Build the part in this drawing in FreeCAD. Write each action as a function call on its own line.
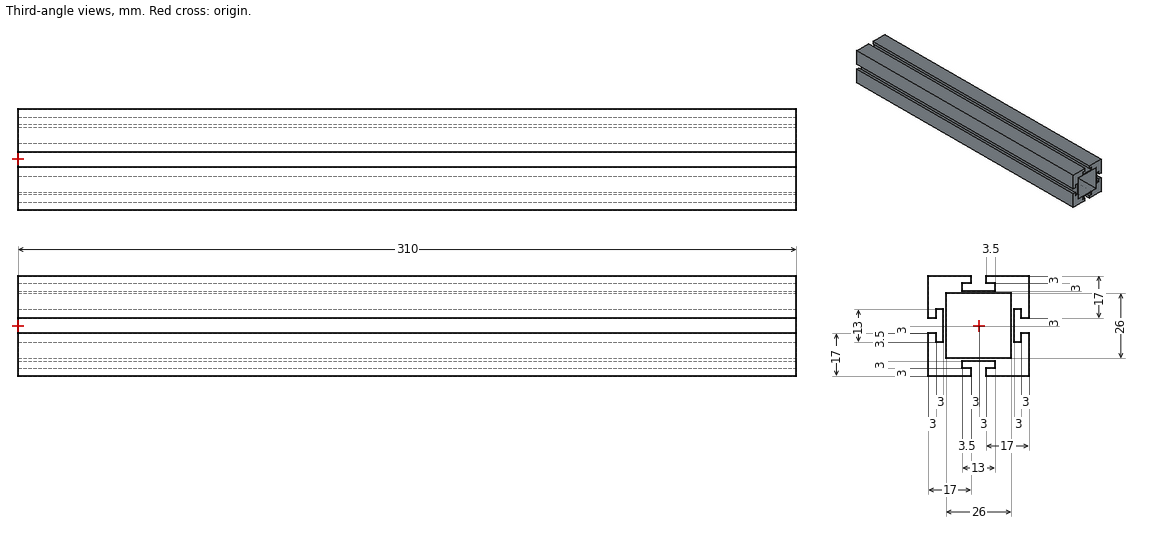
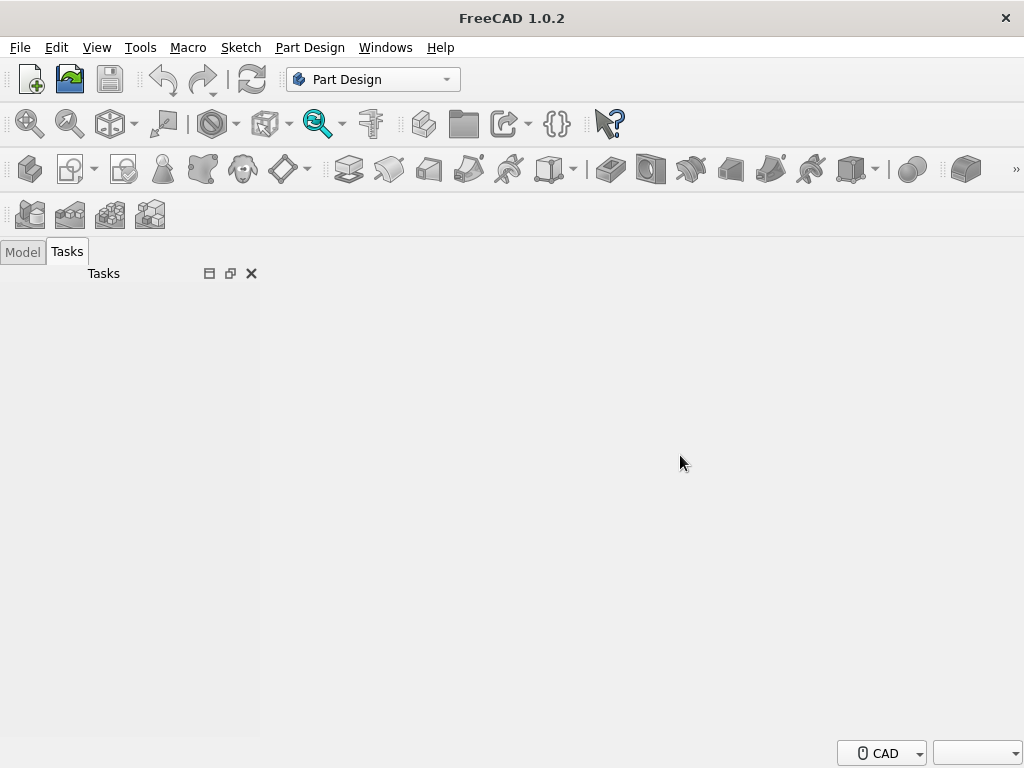
key(ctrl+n)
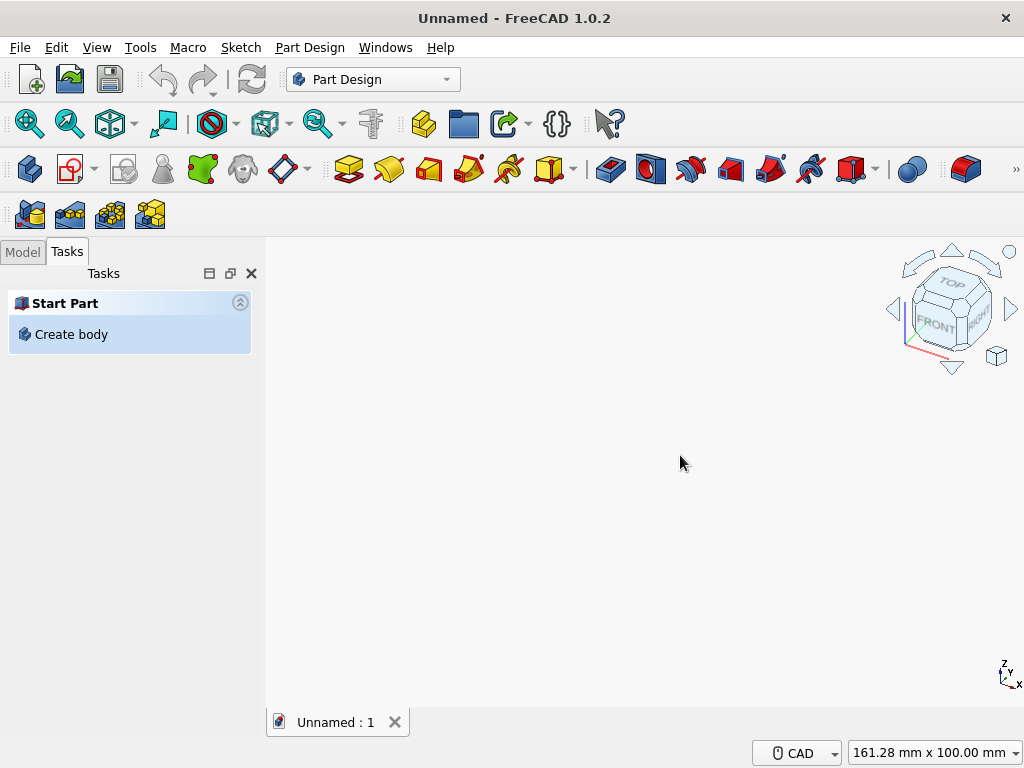
click(70, 170)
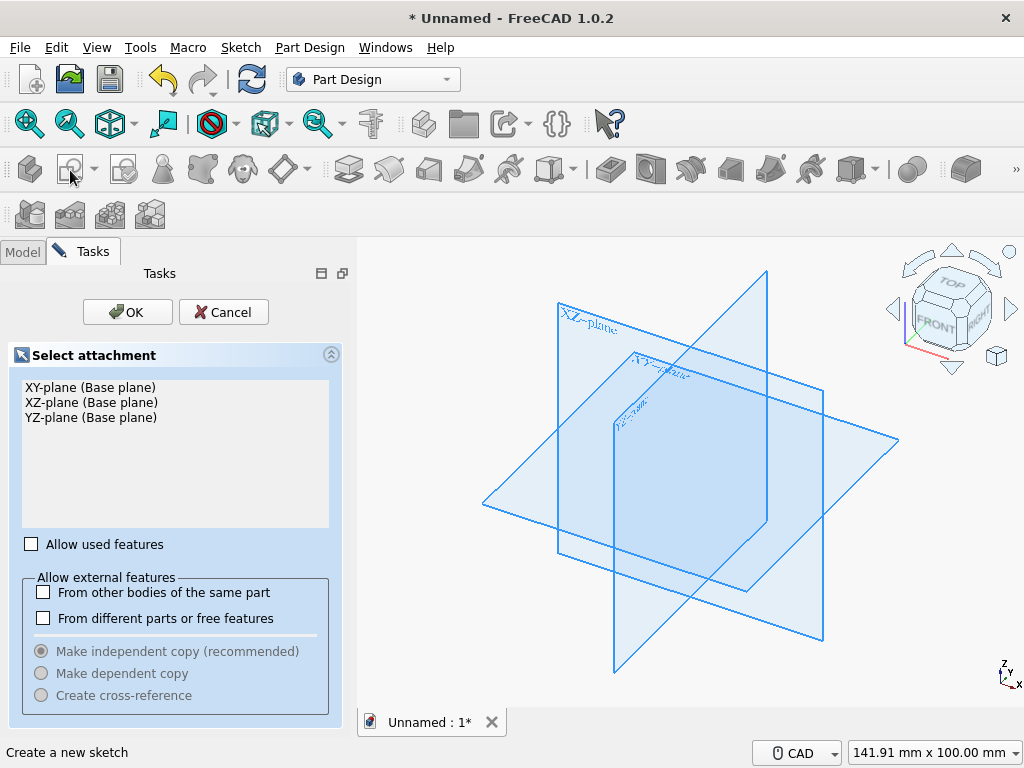
click(82, 418)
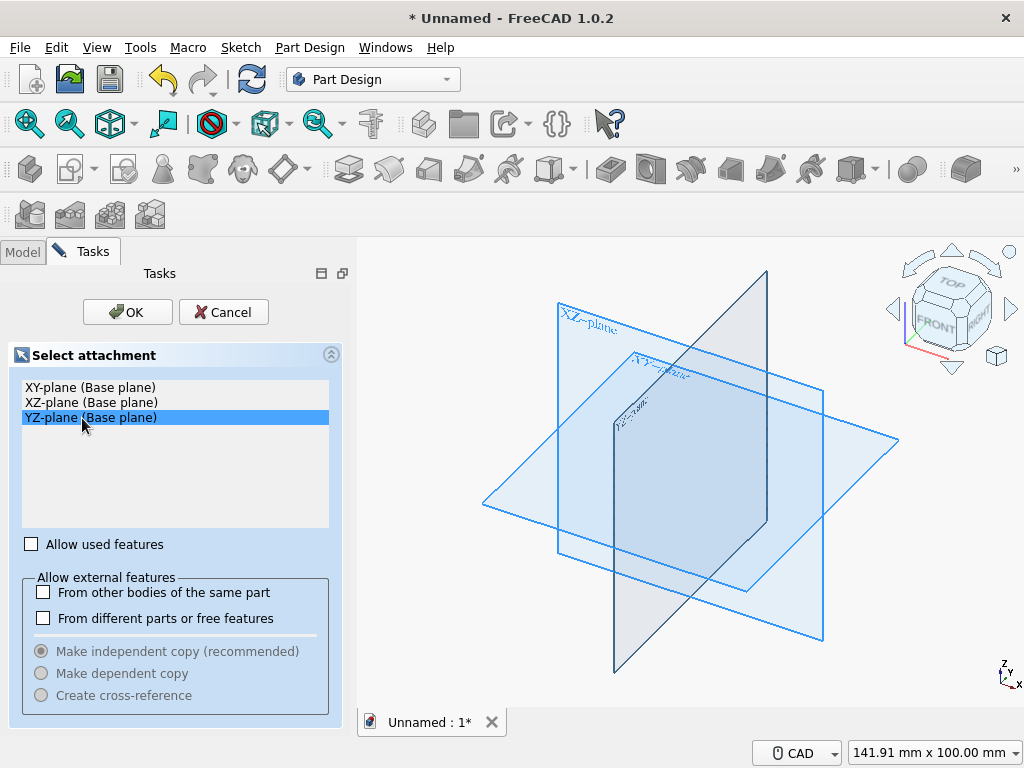
click(128, 312)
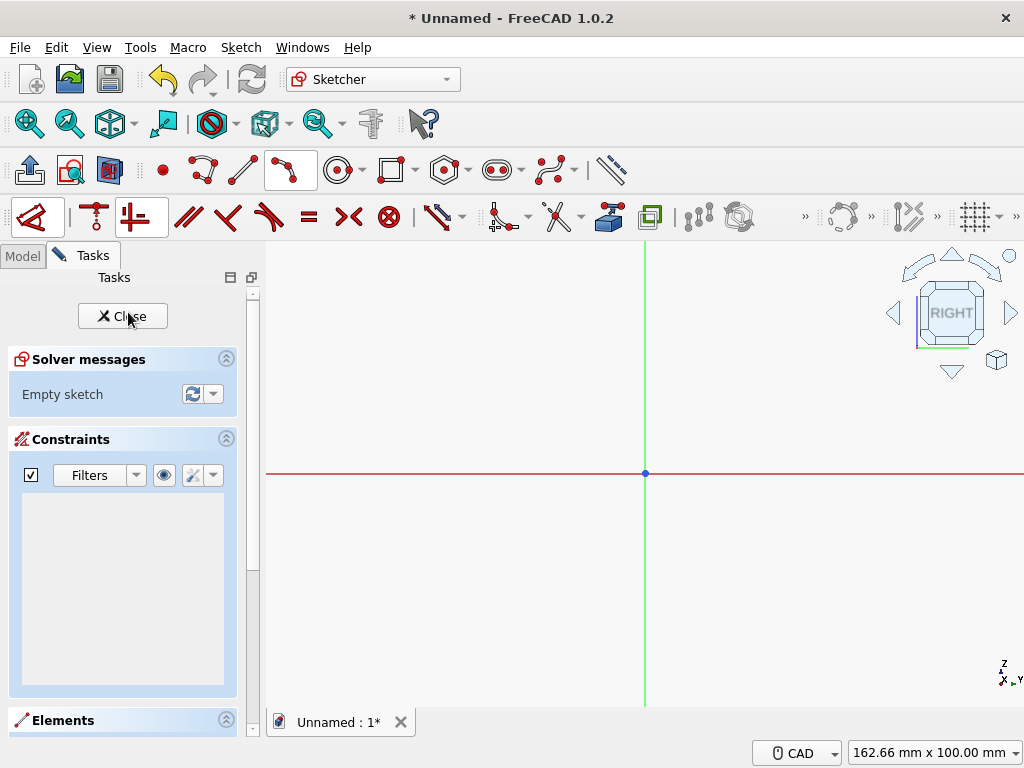
scroll(784, 474, up, 2)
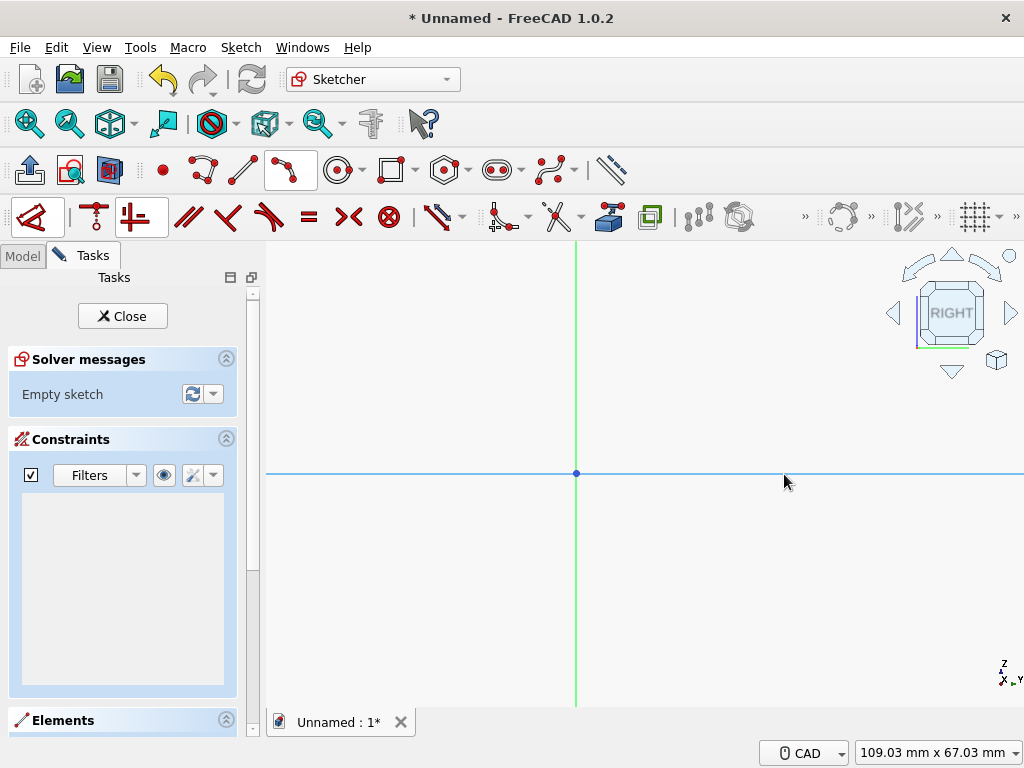
click(204, 170)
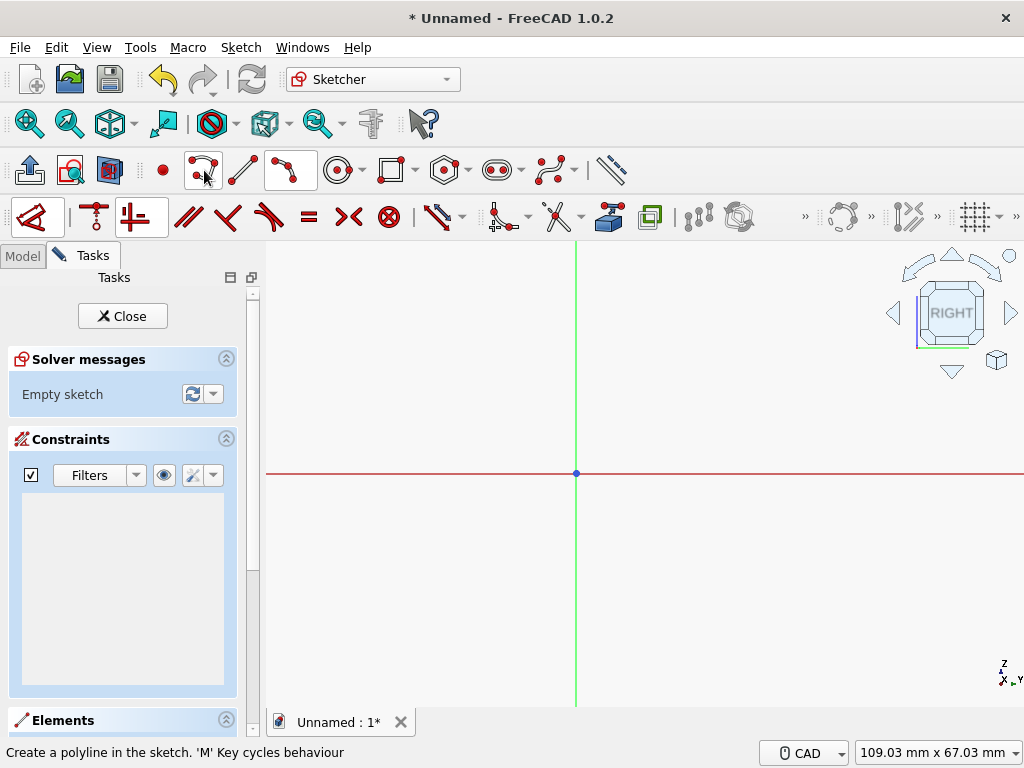
click(479, 429)
click(479, 519)
click(458, 519)
click(458, 495)
click(437, 495)
click(437, 613)
click(555, 613)
click(555, 592)
click(531, 592)
click(531, 571)
click(621, 571)
click(621, 592)
click(597, 592)
click(597, 613)
click(715, 613)
click(715, 495)
click(694, 495)
click(694, 519)
click(674, 519)
click(674, 429)
click(694, 429)
click(694, 453)
click(715, 453)
click(715, 335)
click(597, 335)
click(597, 356)
click(621, 356)
click(621, 376)
click(531, 376)
click(531, 356)
click(555, 356)
click(555, 335)
click(437, 335)
click(437, 453)
click(458, 453)
click(458, 429)
click(479, 430)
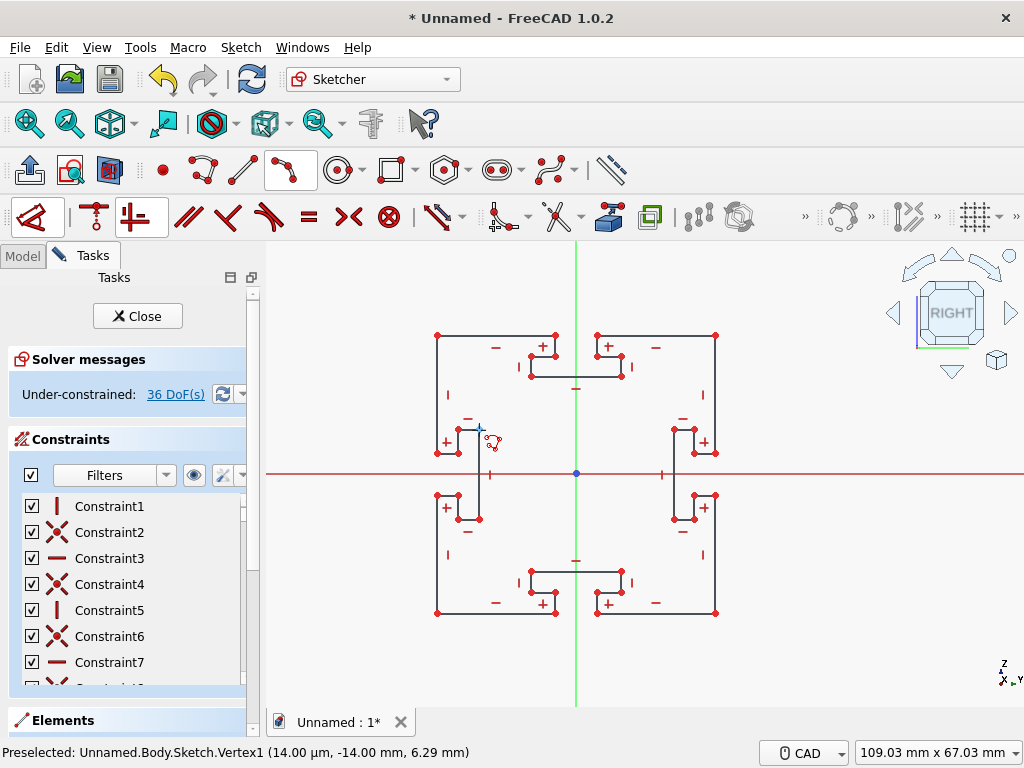
click(418, 170)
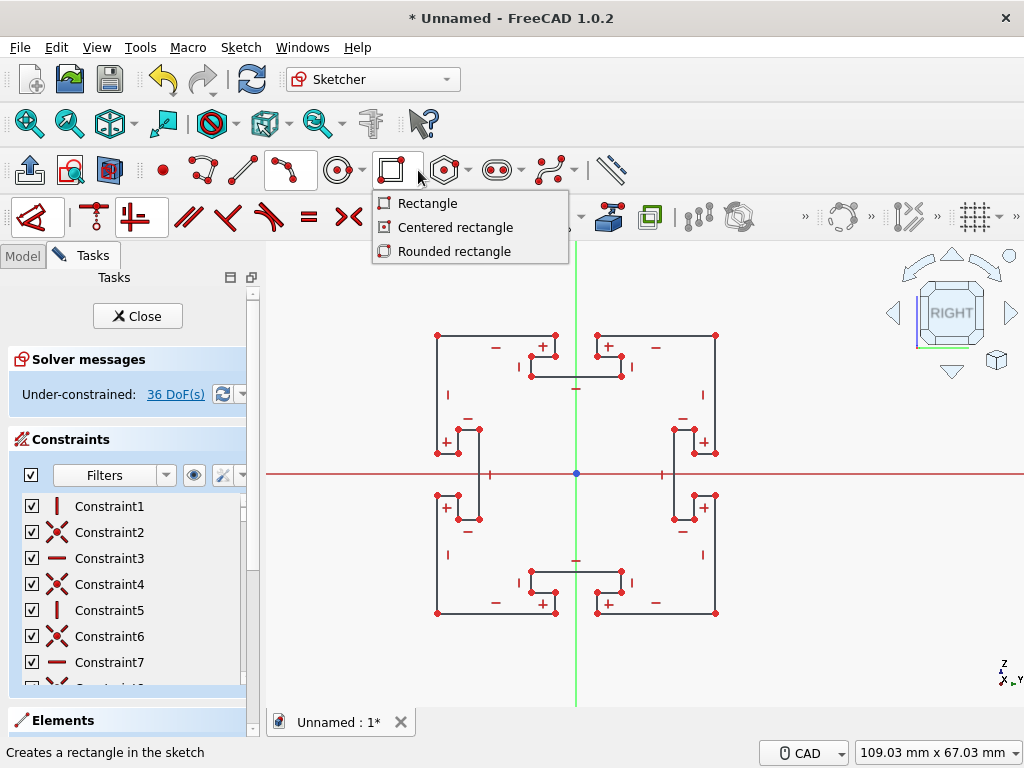
click(470, 227)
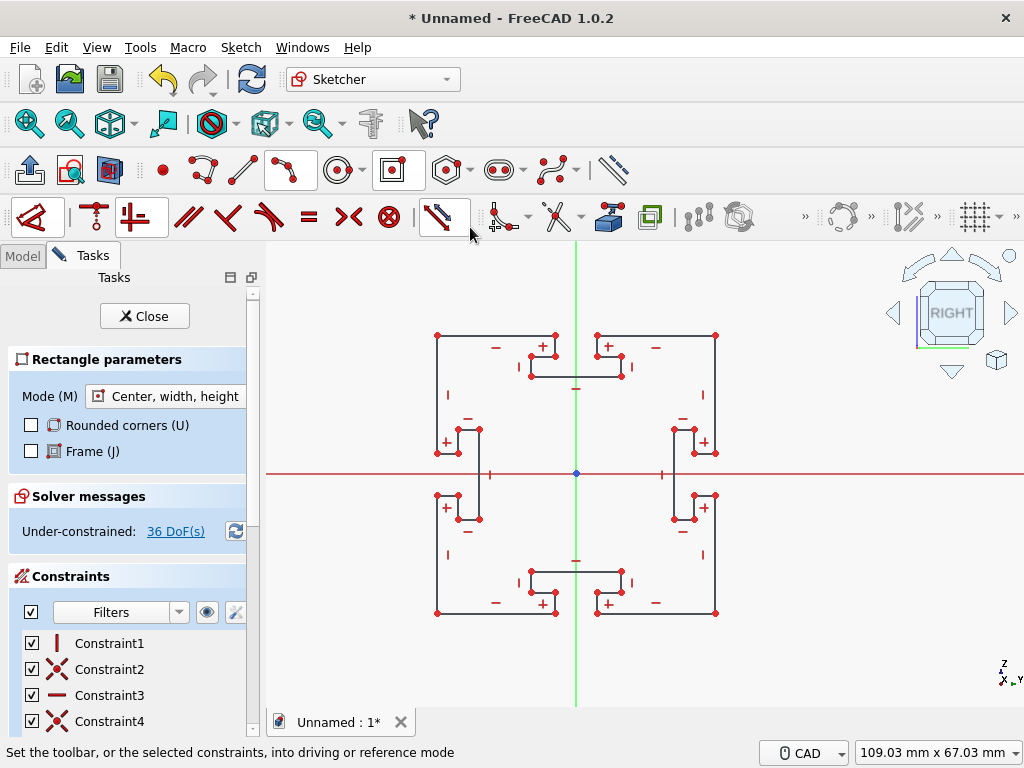
click(576, 474)
click(667, 383)
key(Escape)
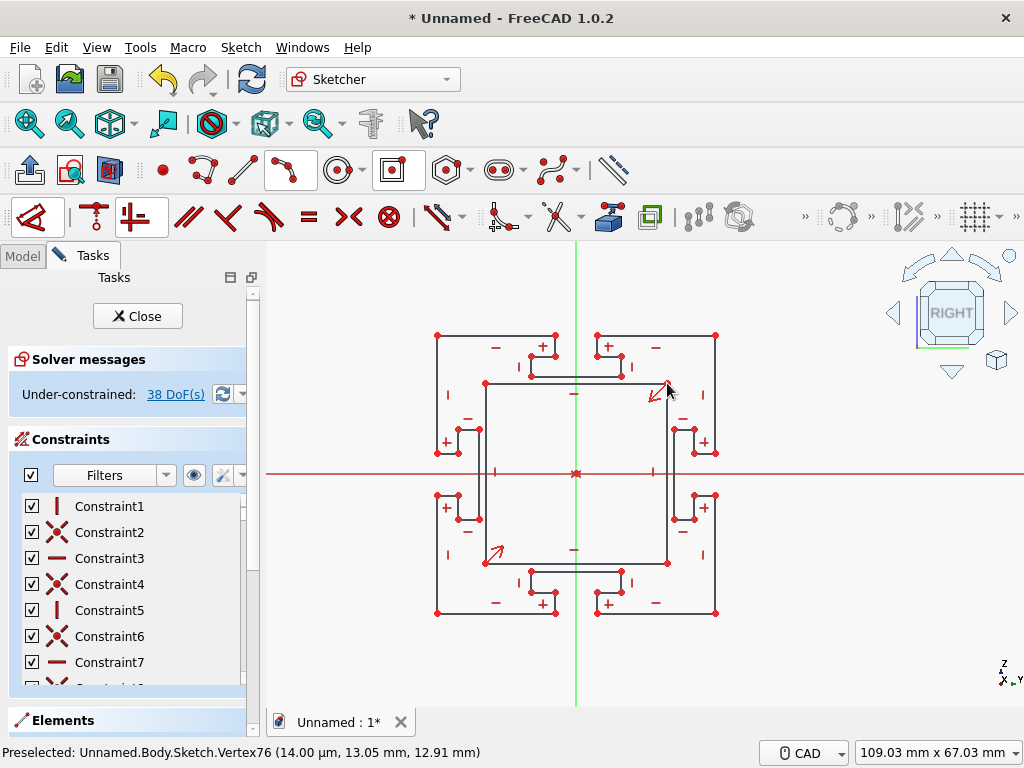
click(32, 218)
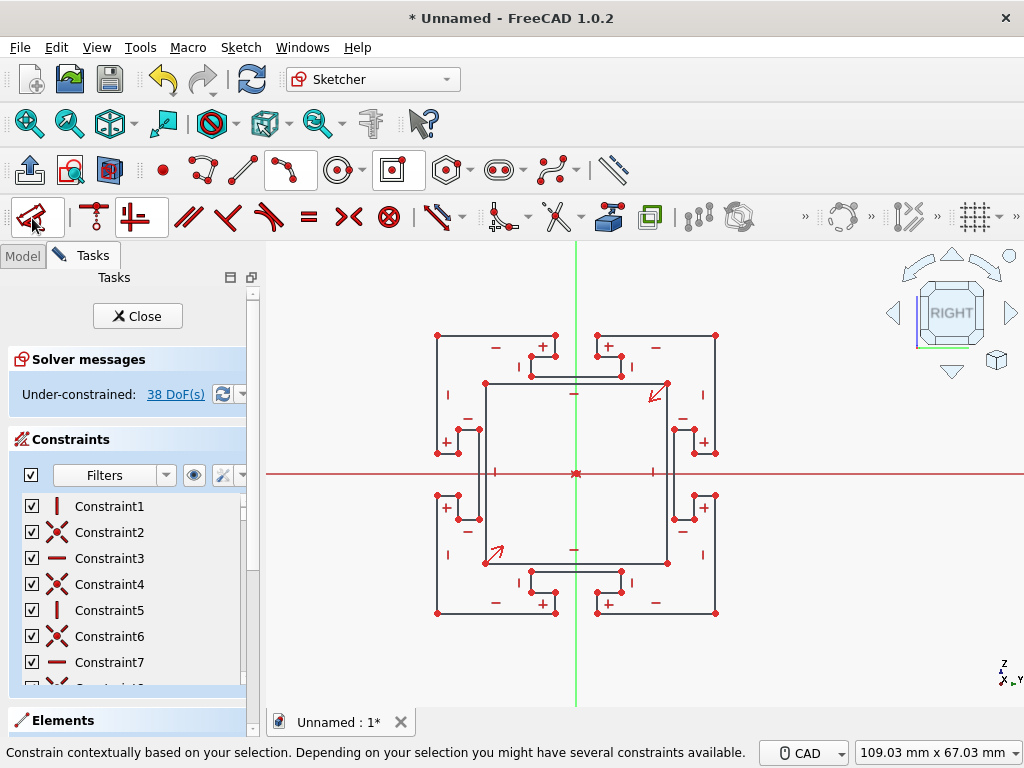
scroll(469, 520, up, 4)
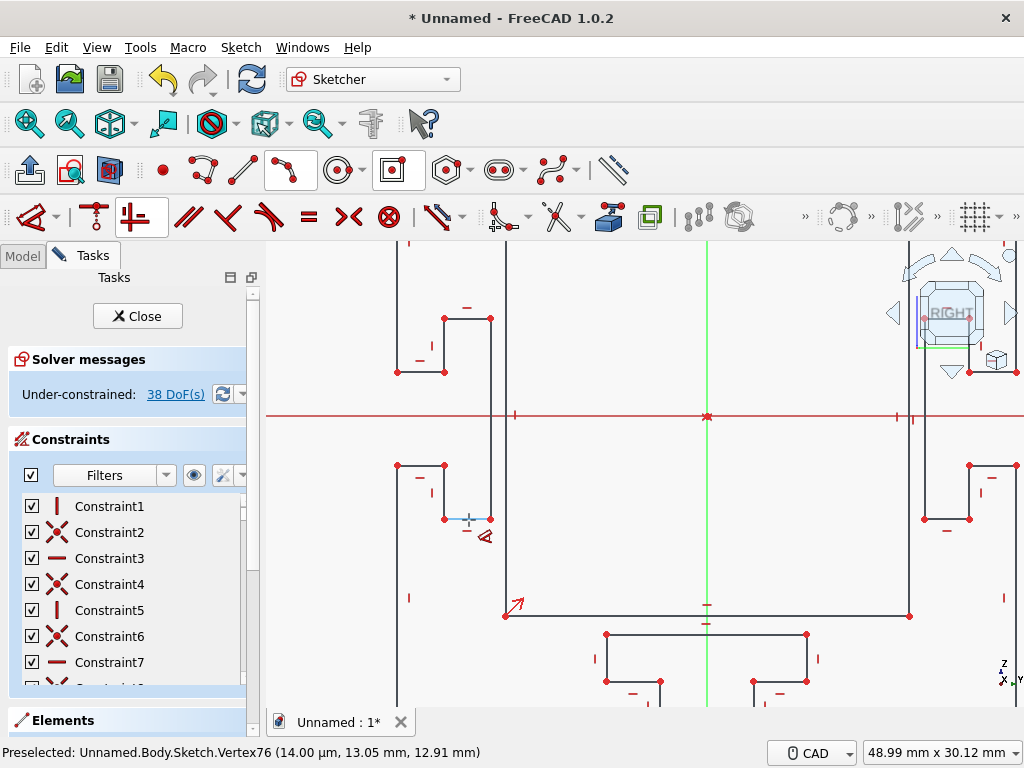
click(468, 519)
click(468, 553)